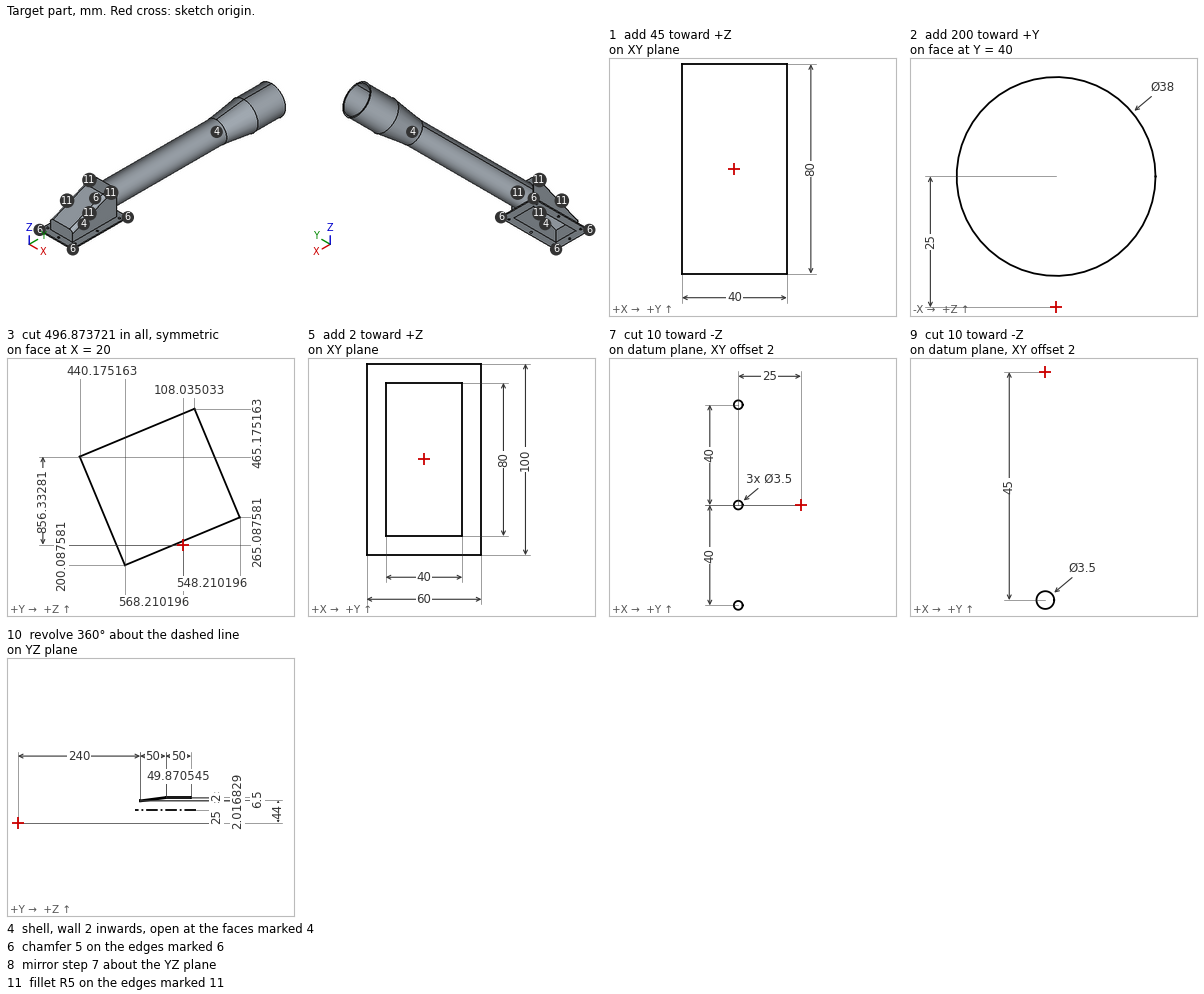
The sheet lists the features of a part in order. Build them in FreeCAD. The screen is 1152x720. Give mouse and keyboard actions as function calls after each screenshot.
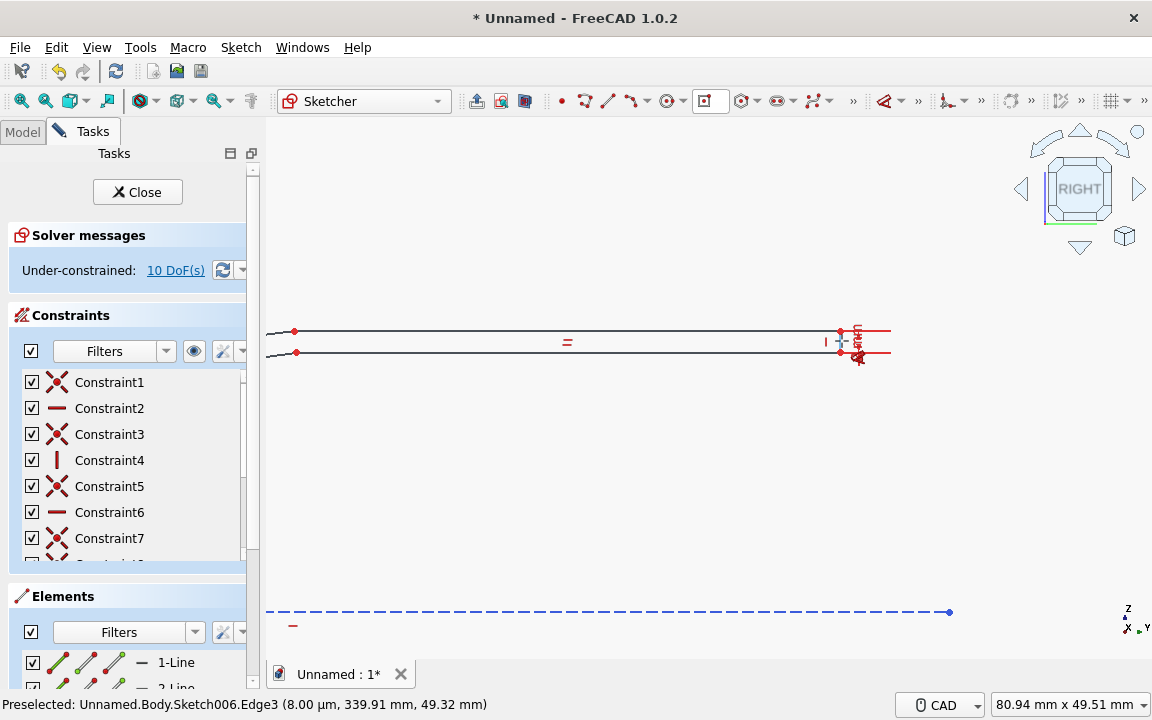
scroll(781, 338, up, 3)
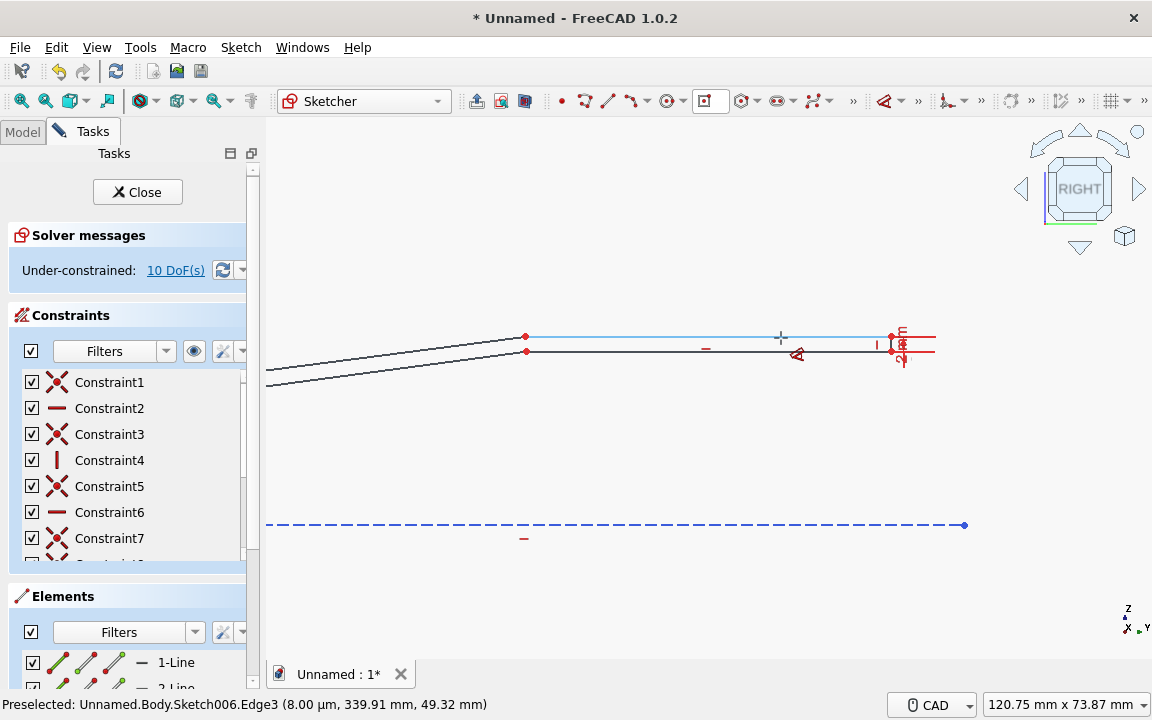
click(781, 337)
click(708, 303)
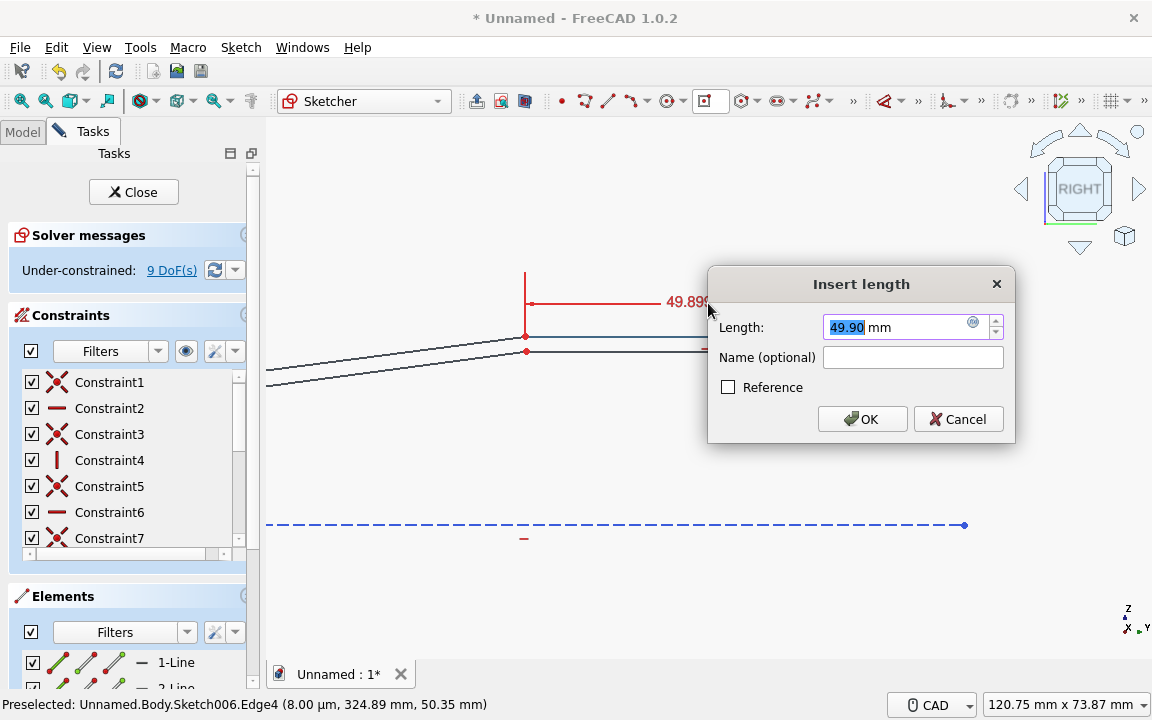
text(50)
key(Return)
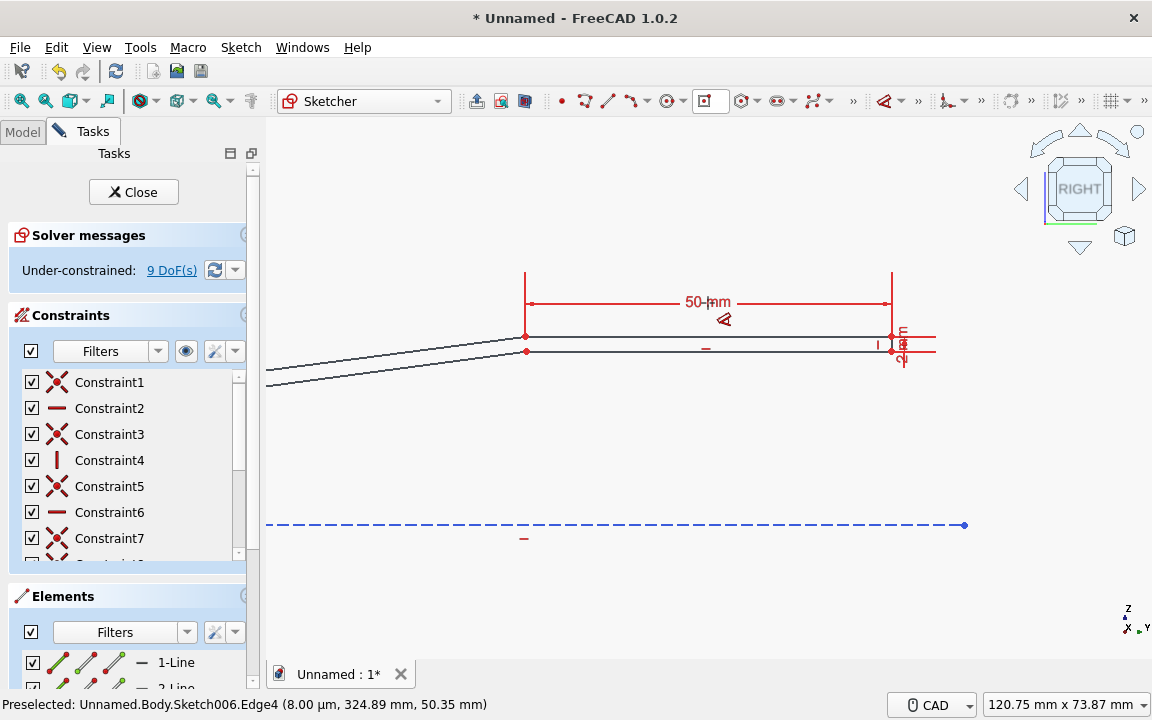
scroll(781, 338, down, 3)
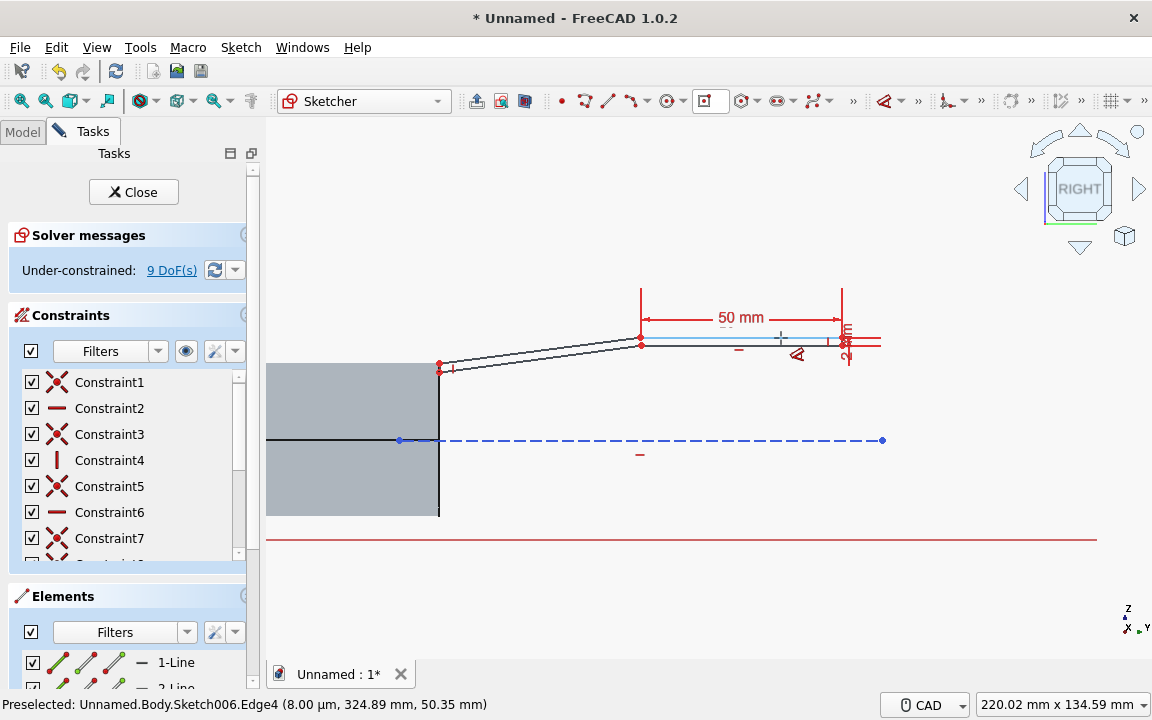
scroll(440, 364, up, 2)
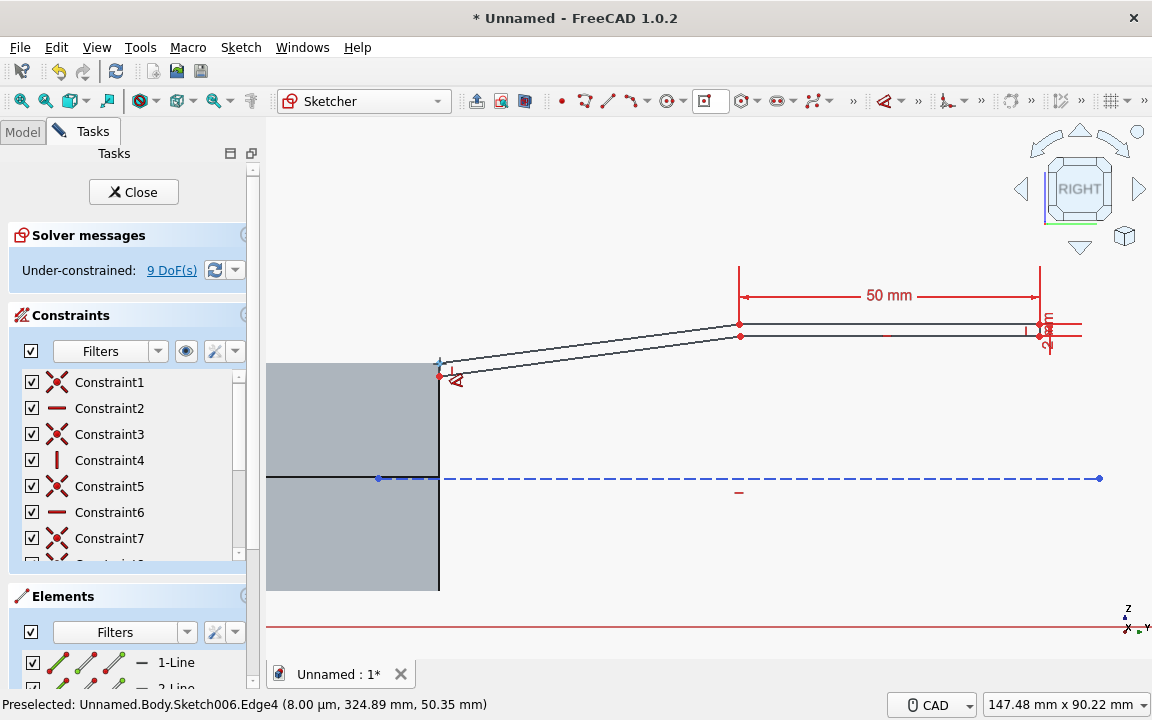
click(439, 363)
click(473, 495)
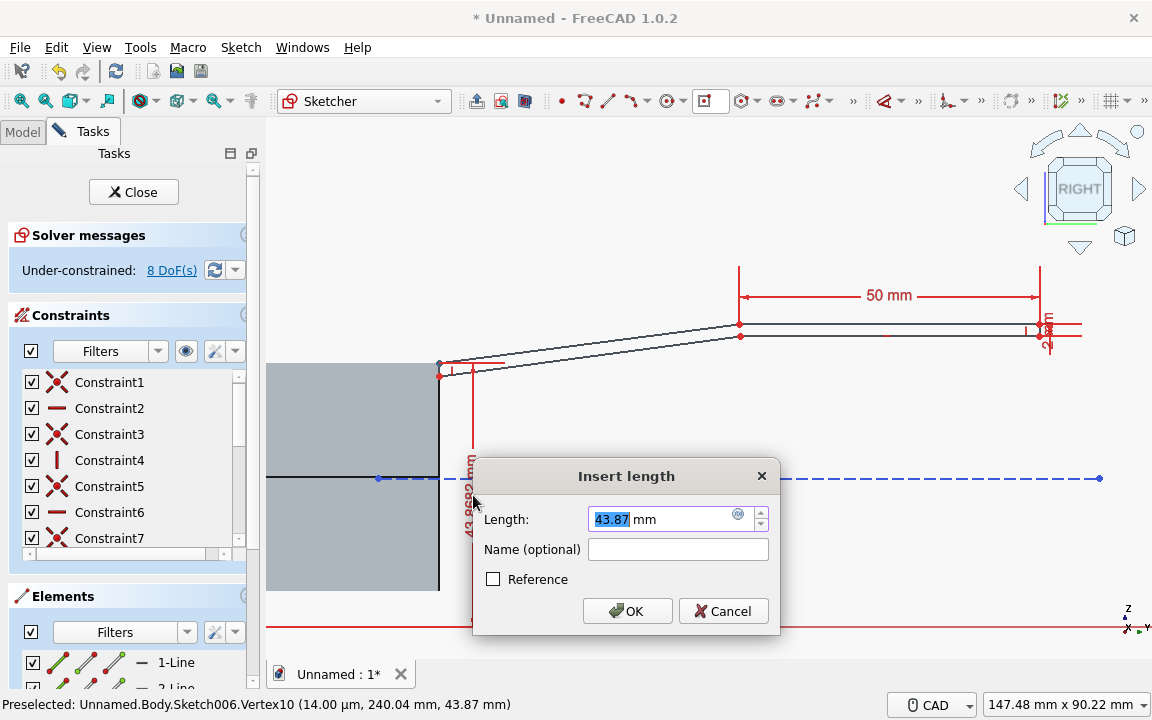
text(44)
key(Return)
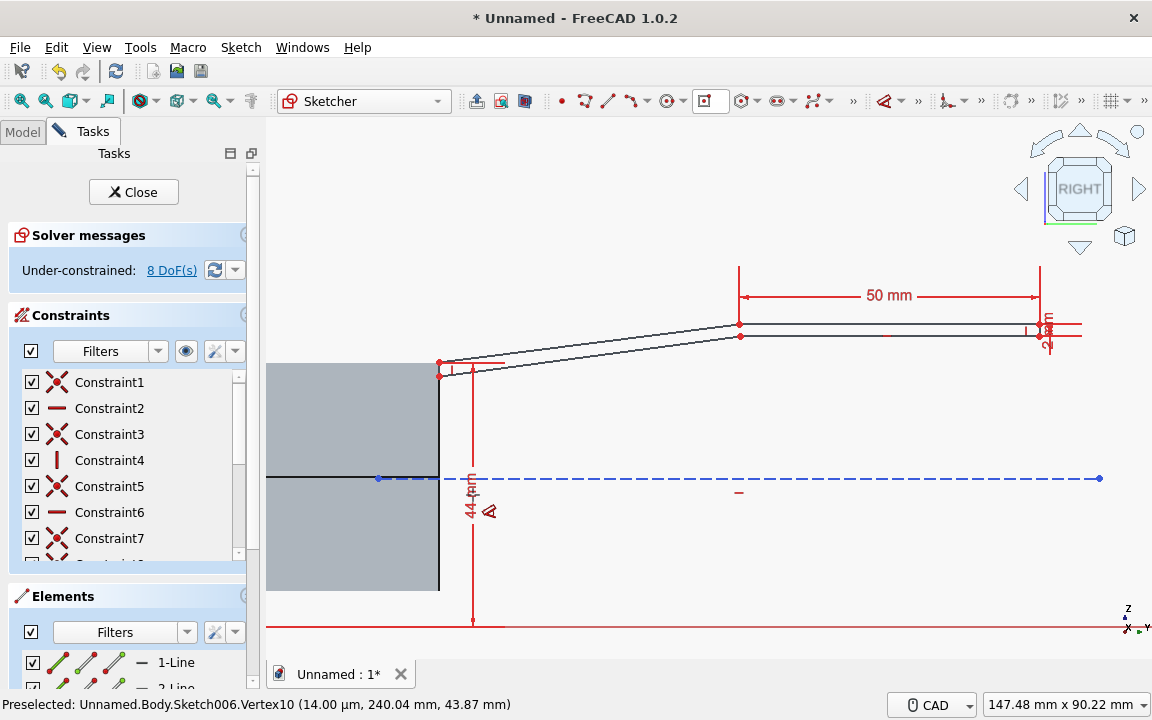
scroll(439, 363, down, 2)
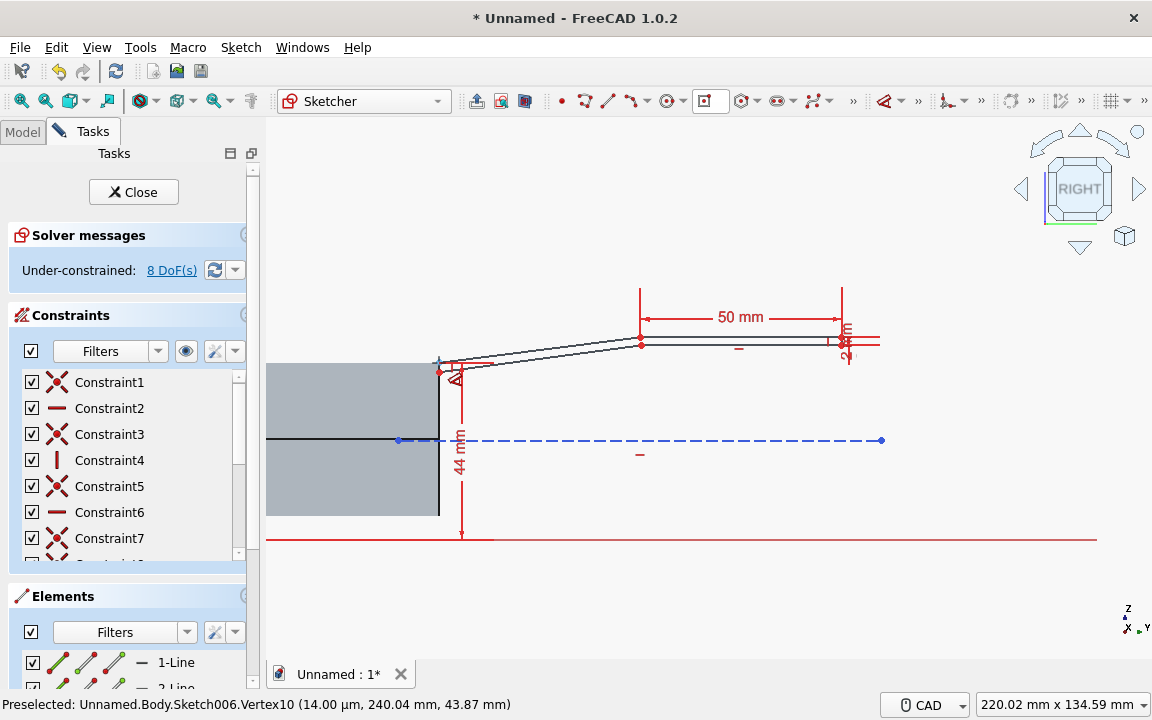
click(882, 441)
click(916, 490)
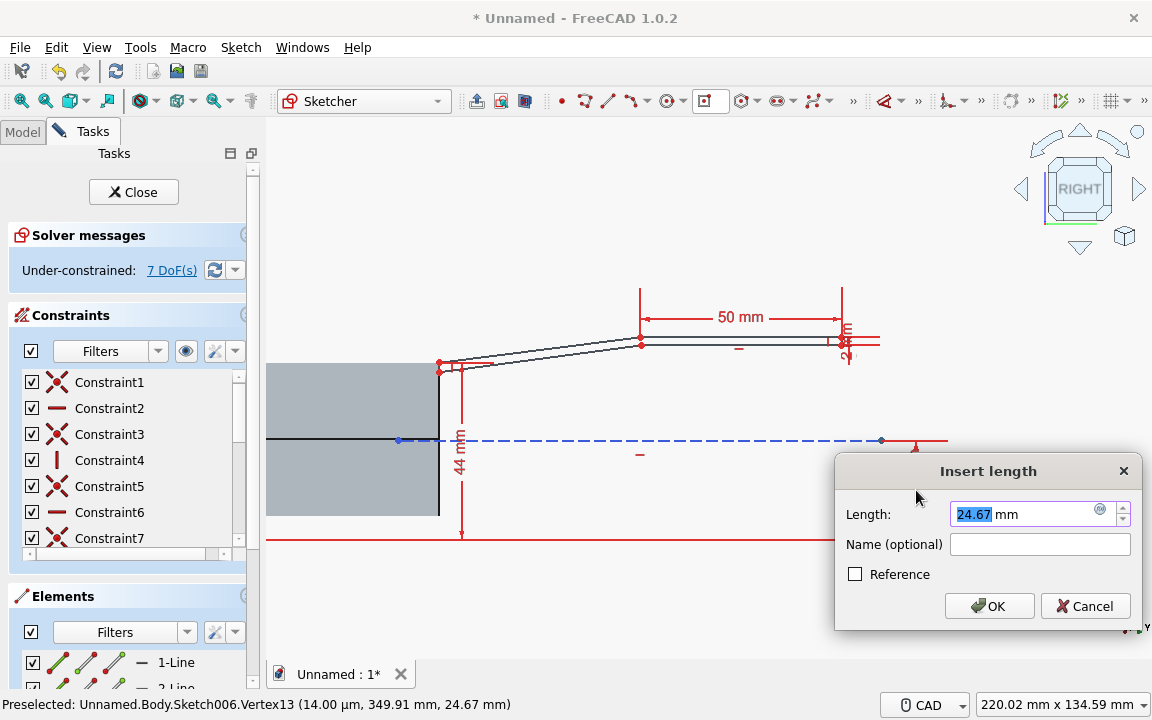
text(25)
key(Return)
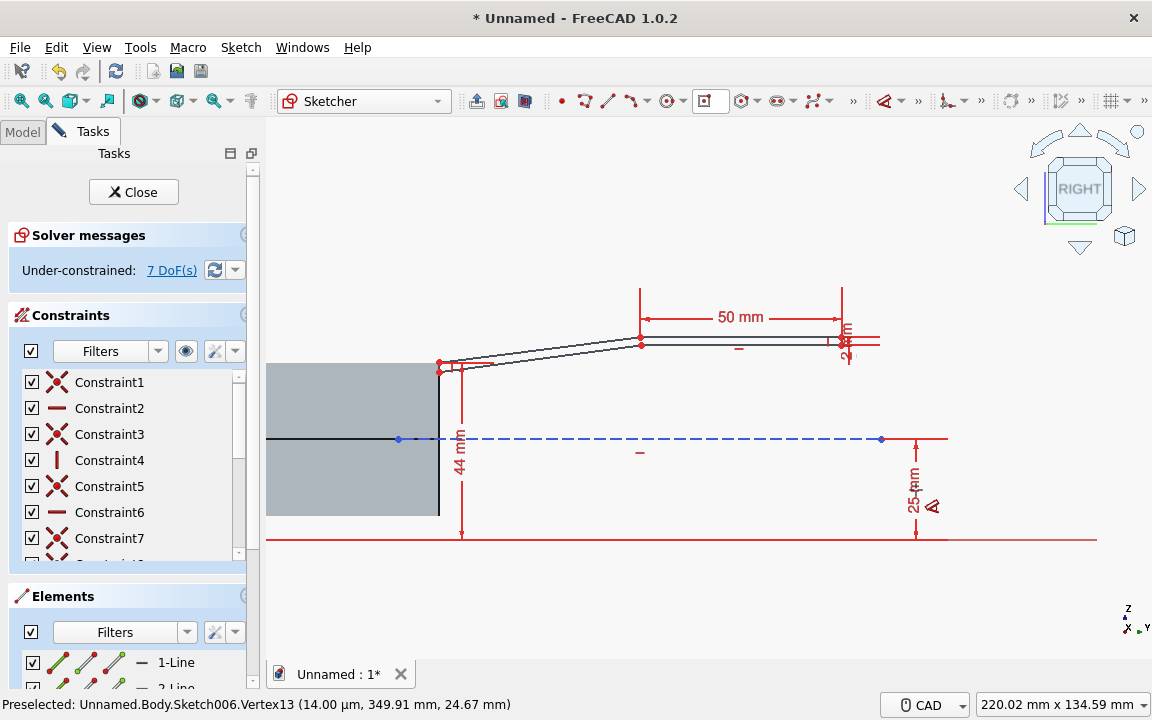
scroll(500, 355, up, 3)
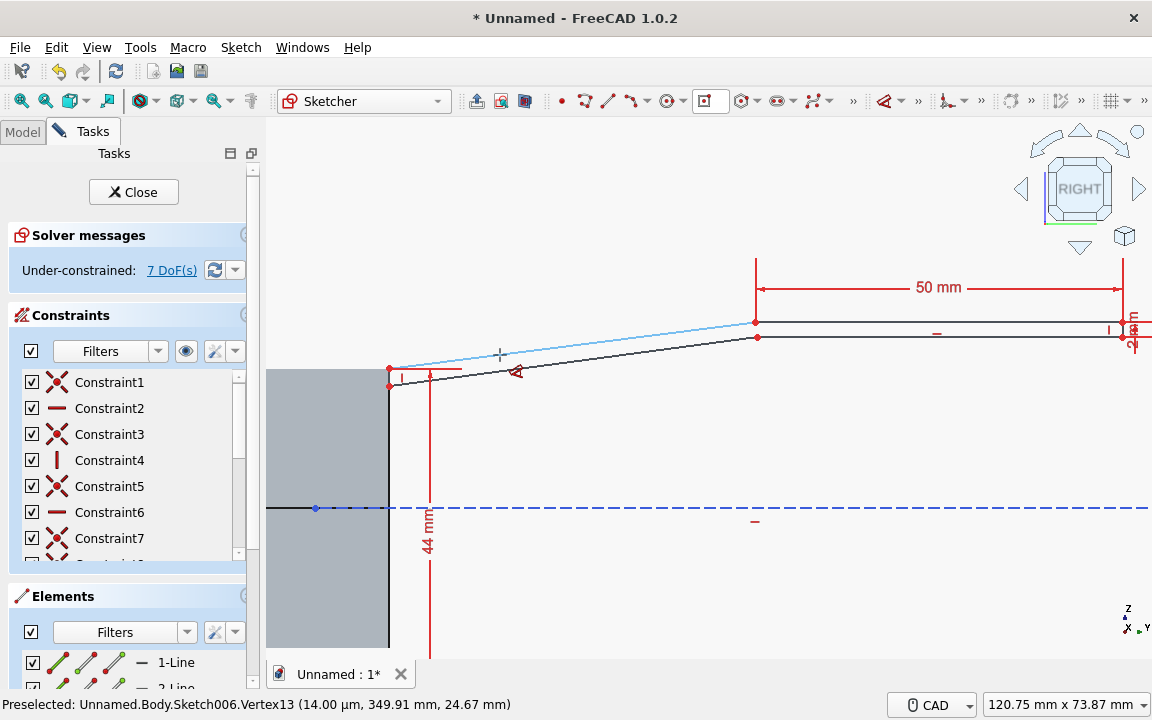
click(499, 355)
click(572, 288)